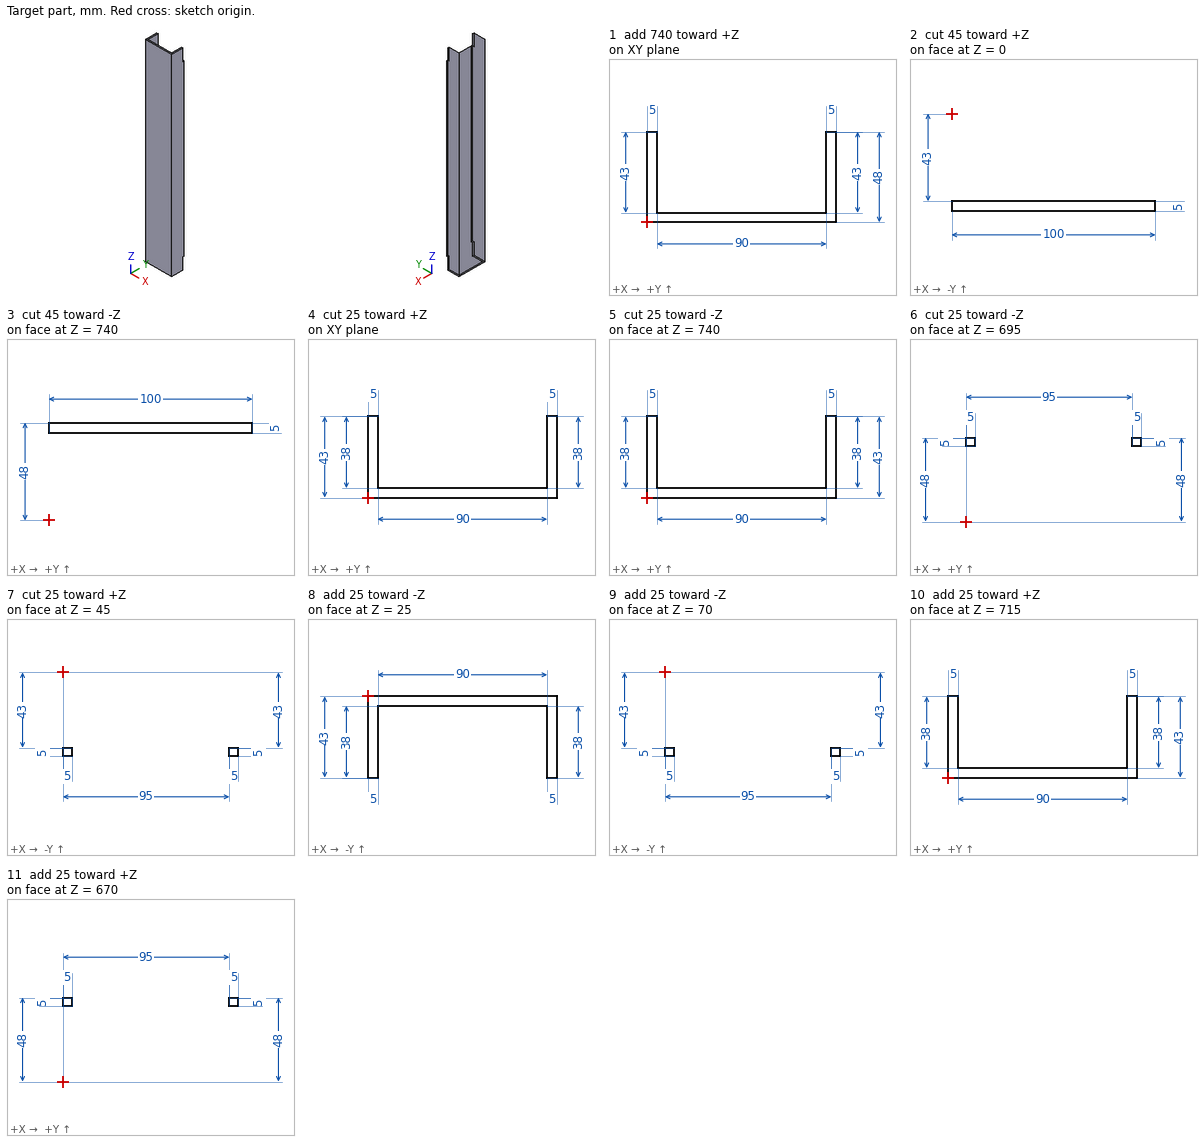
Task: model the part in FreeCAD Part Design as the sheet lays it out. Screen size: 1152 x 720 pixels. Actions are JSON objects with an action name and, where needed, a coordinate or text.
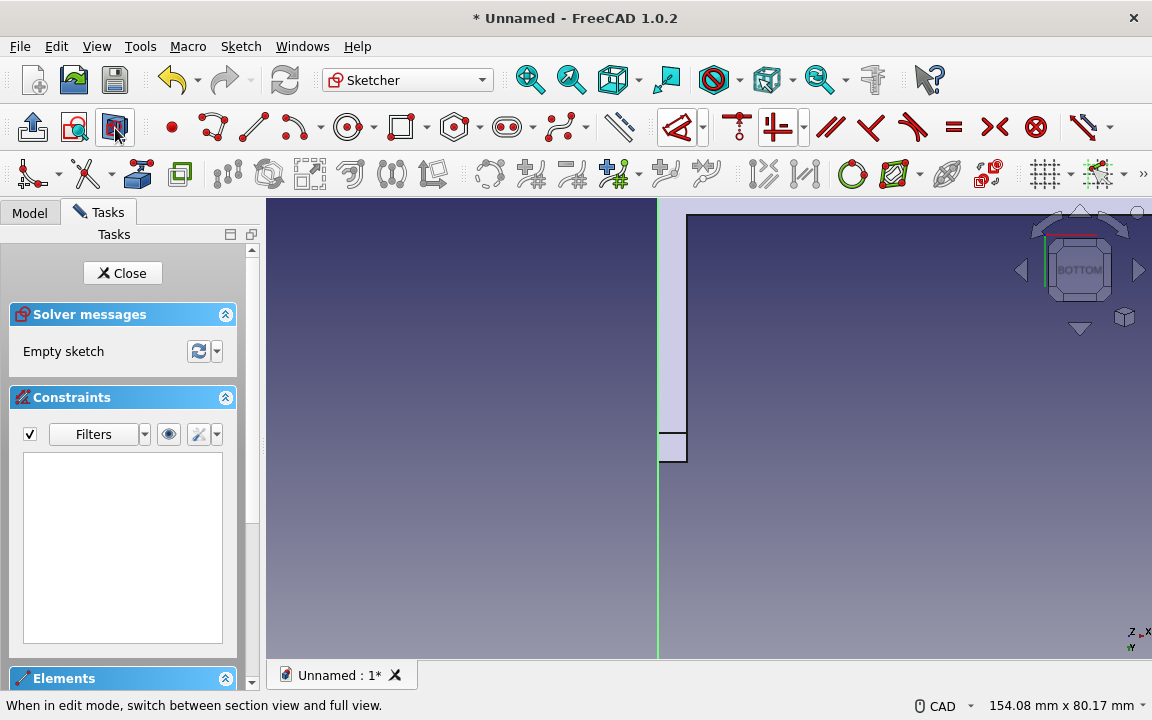
{"action": "scroll", "coordinate": [294, 631], "scroll_direction": "down", "scroll_amount": 2}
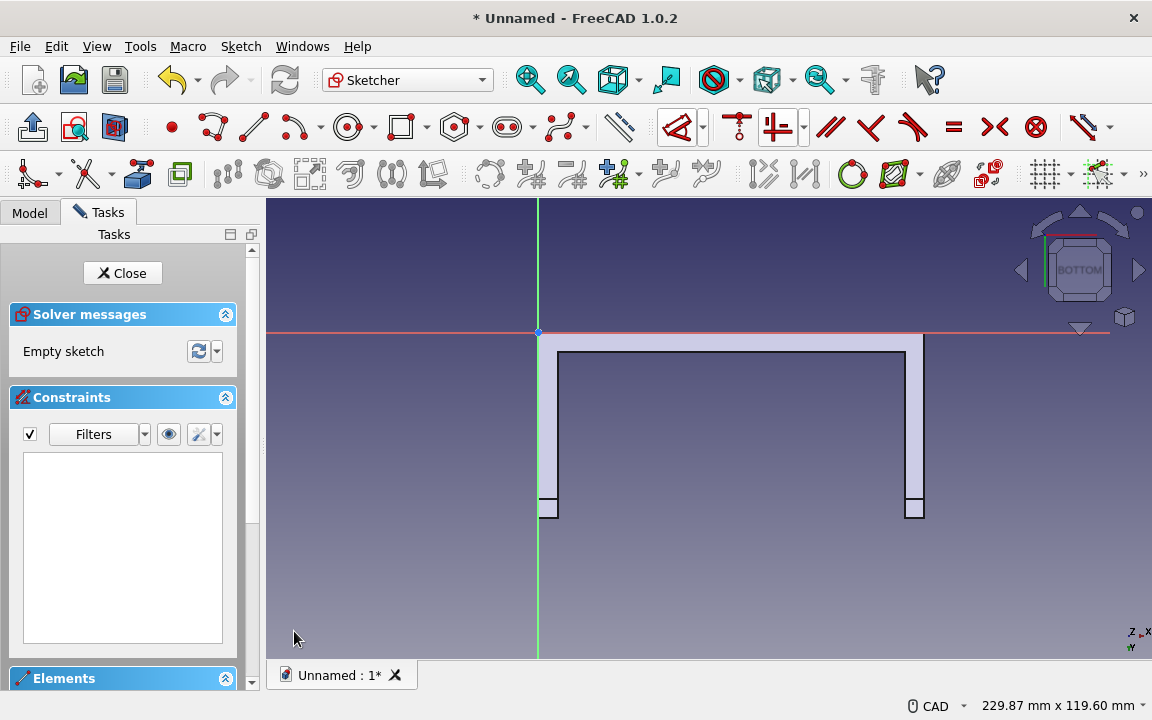
{"action": "left_click", "coordinate": [400, 128]}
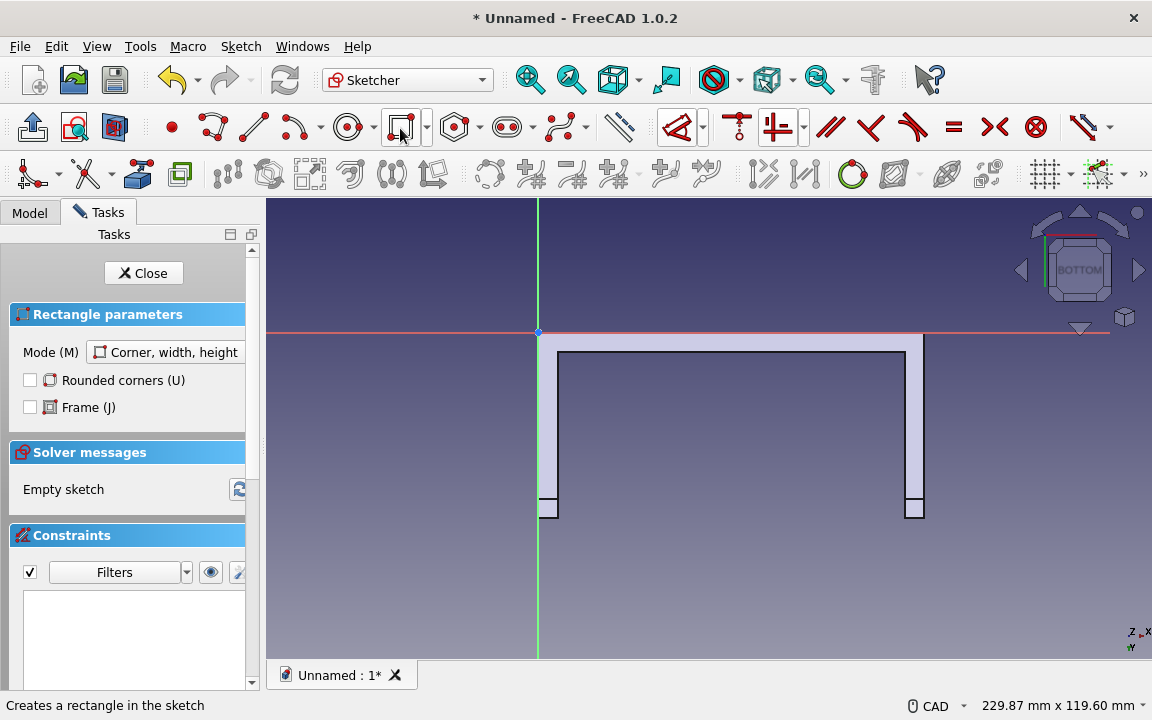
{"action": "left_click", "coordinate": [538, 499]}
{"action": "mouse_move", "coordinate": [558, 518]}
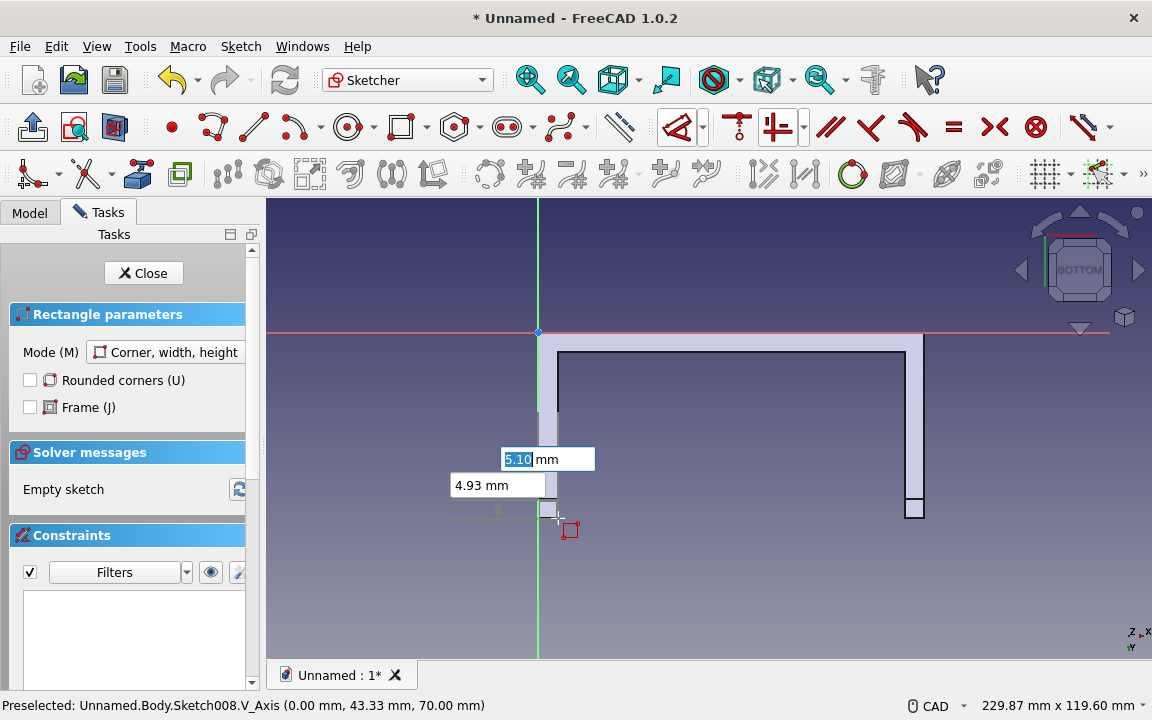
{"action": "type", "text": "5"}
{"action": "key", "text": "Tab"}
{"action": "type", "text": "5"}
{"action": "key", "text": "Return"}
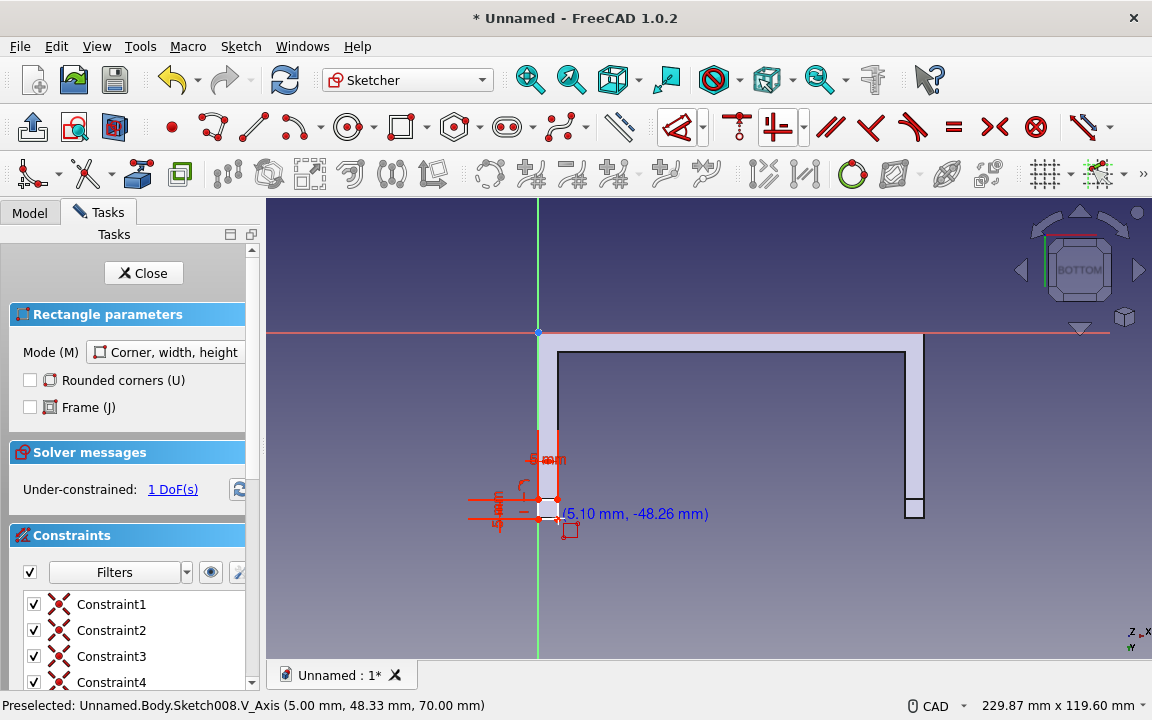
{"action": "left_click", "coordinate": [905, 499]}
{"action": "mouse_move", "coordinate": [924, 518]}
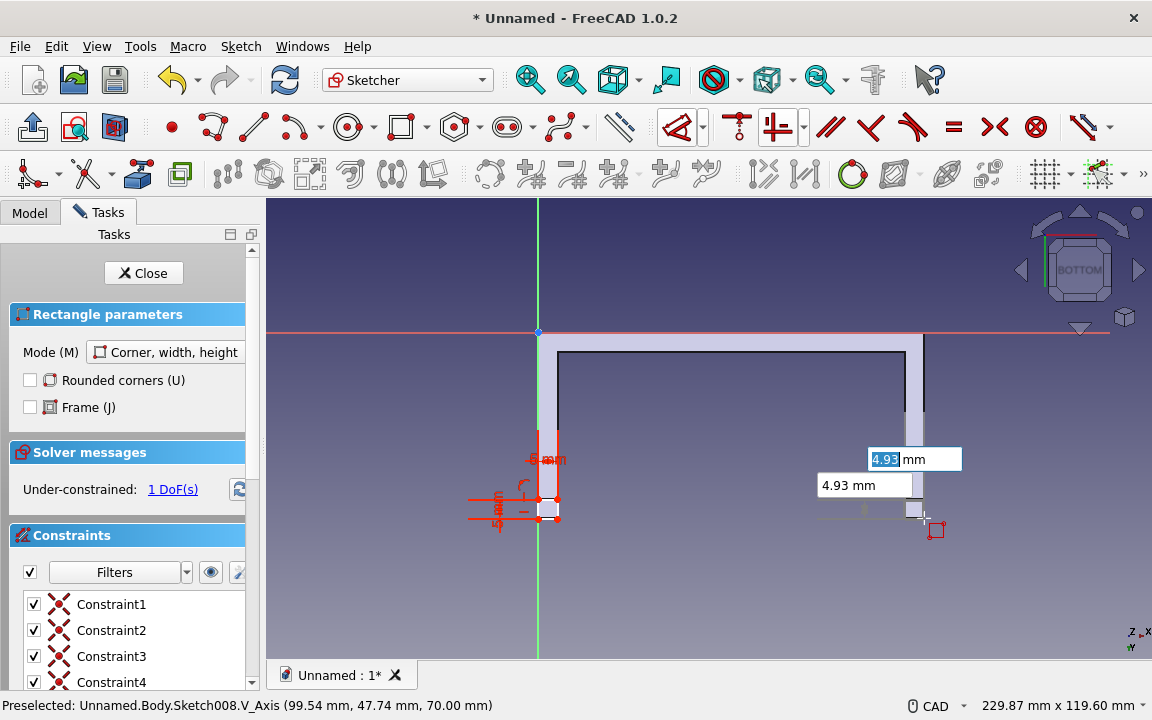
{"action": "type", "text": "5"}
{"action": "key", "text": "Tab"}
{"action": "type", "text": "5"}
{"action": "key", "text": "Return"}
{"action": "key", "text": "Escape"}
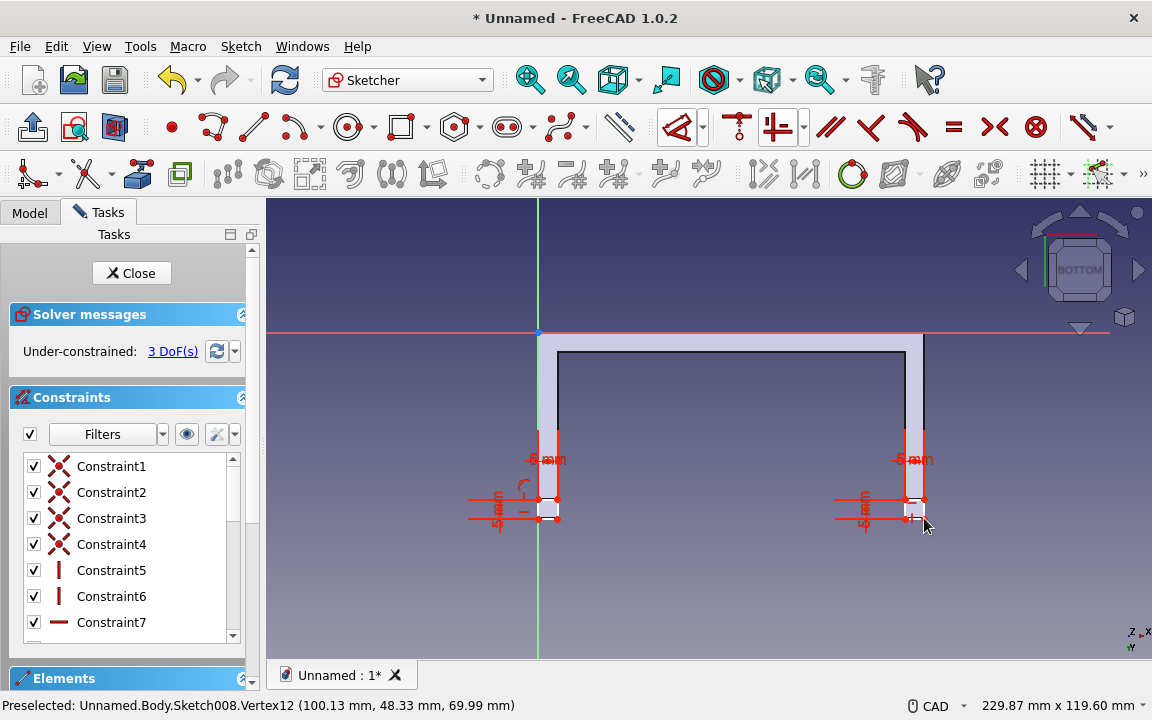
{"action": "left_click", "coordinate": [538, 500]}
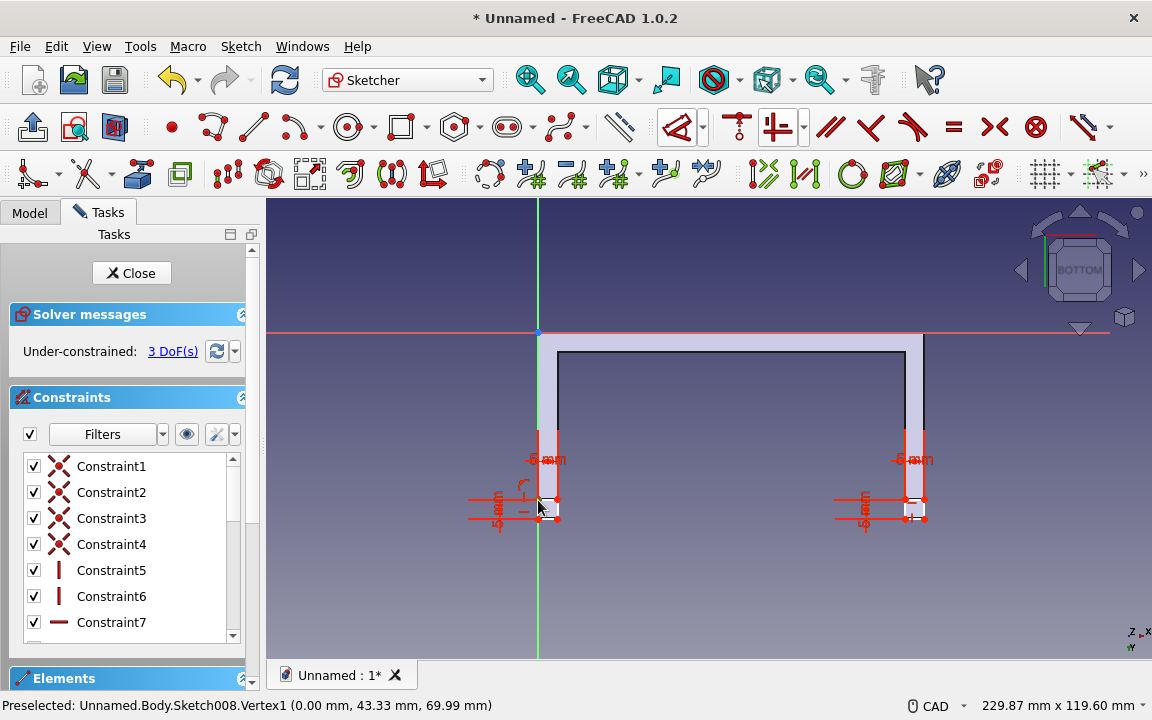
{"action": "left_click", "coordinate": [702, 128]}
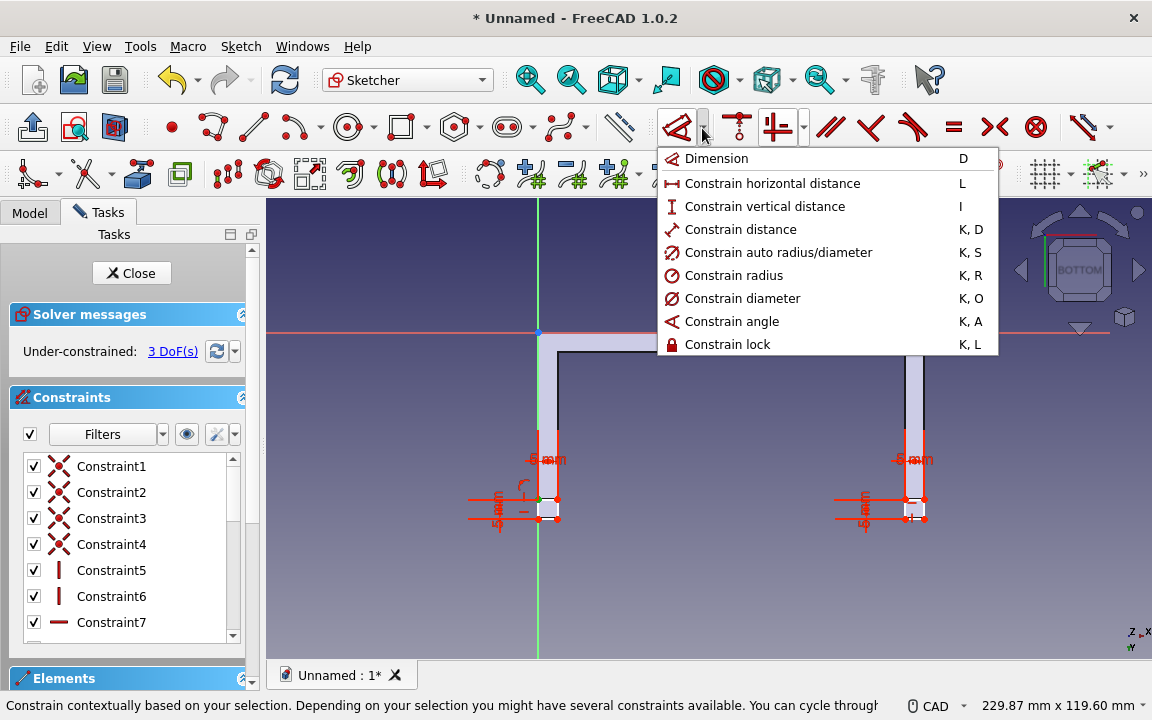
{"action": "left_click", "coordinate": [828, 206]}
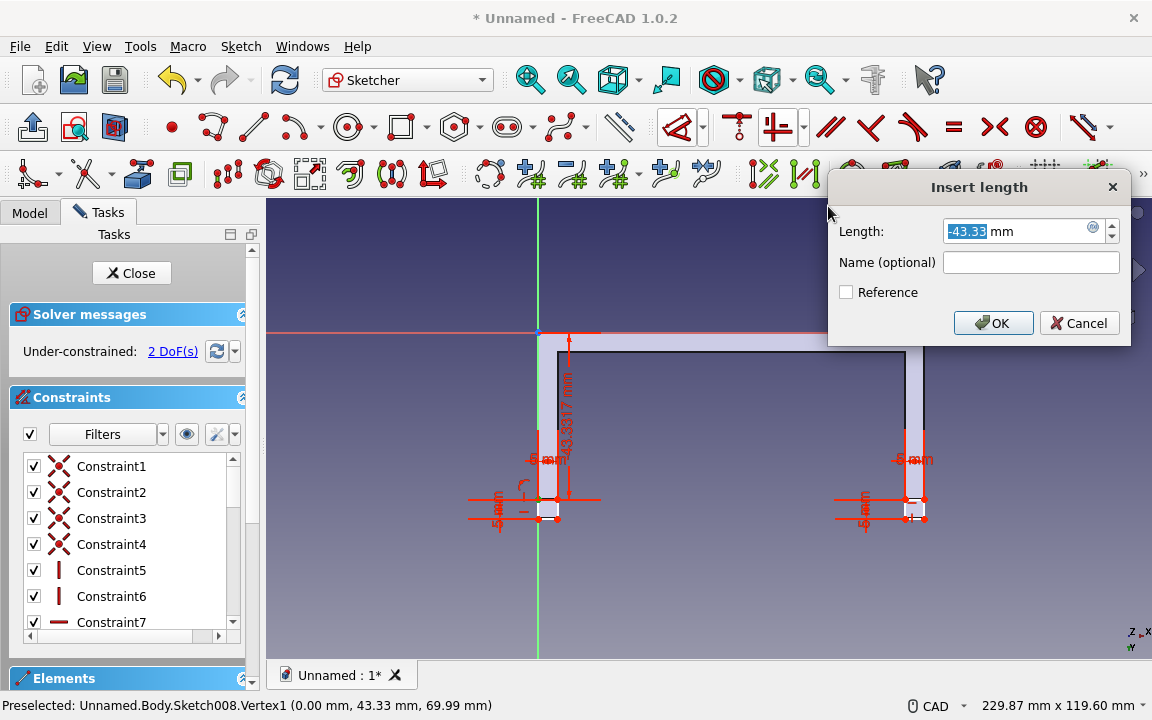
{"action": "type", "text": "-43"}
{"action": "key", "text": "Return"}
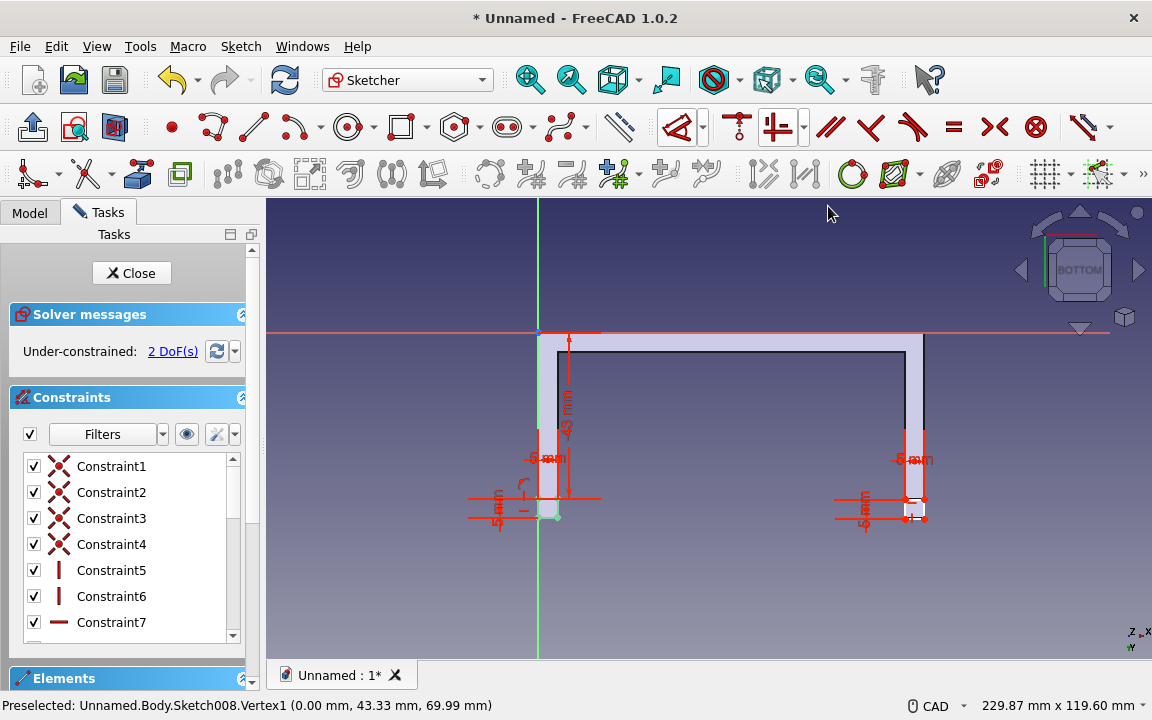
{"action": "left_click", "coordinate": [905, 500]}